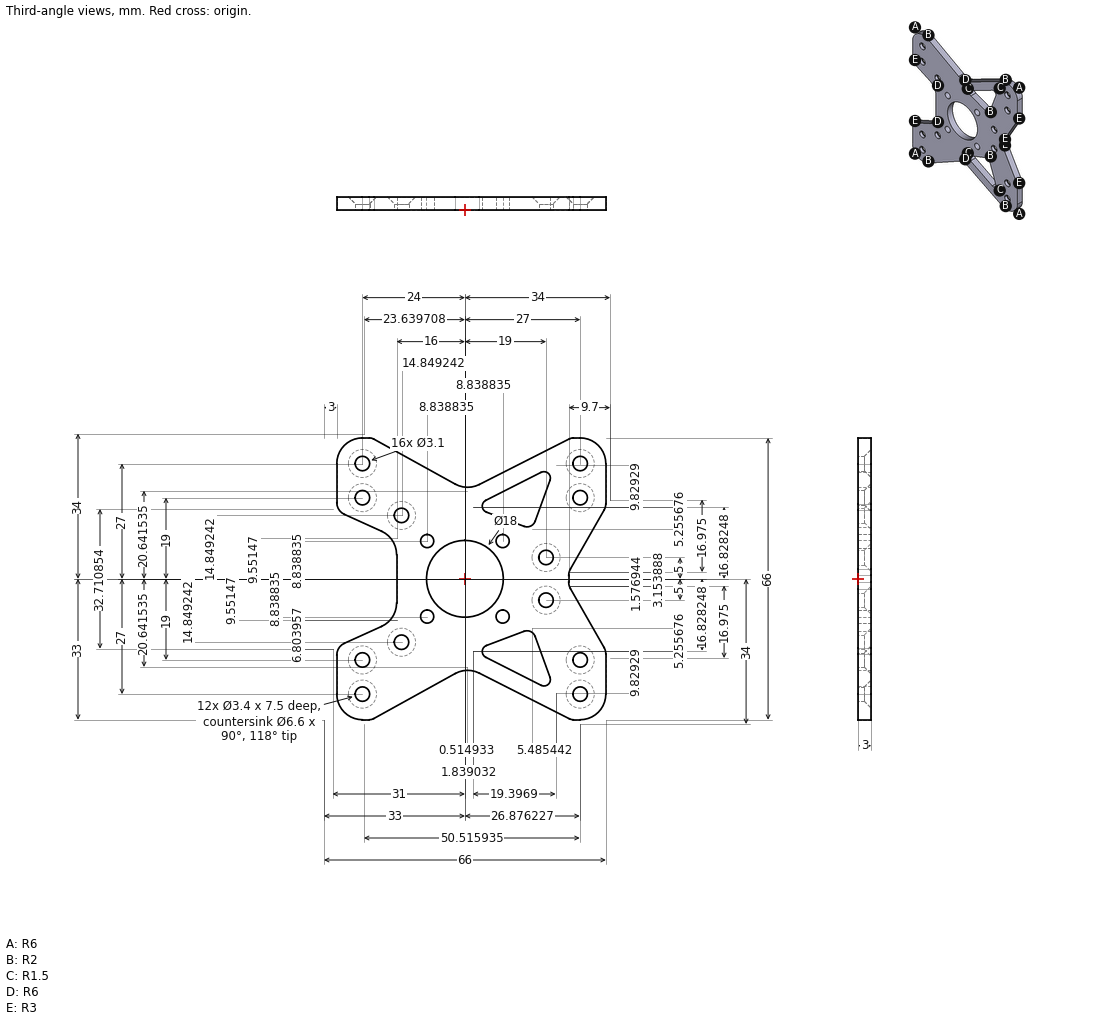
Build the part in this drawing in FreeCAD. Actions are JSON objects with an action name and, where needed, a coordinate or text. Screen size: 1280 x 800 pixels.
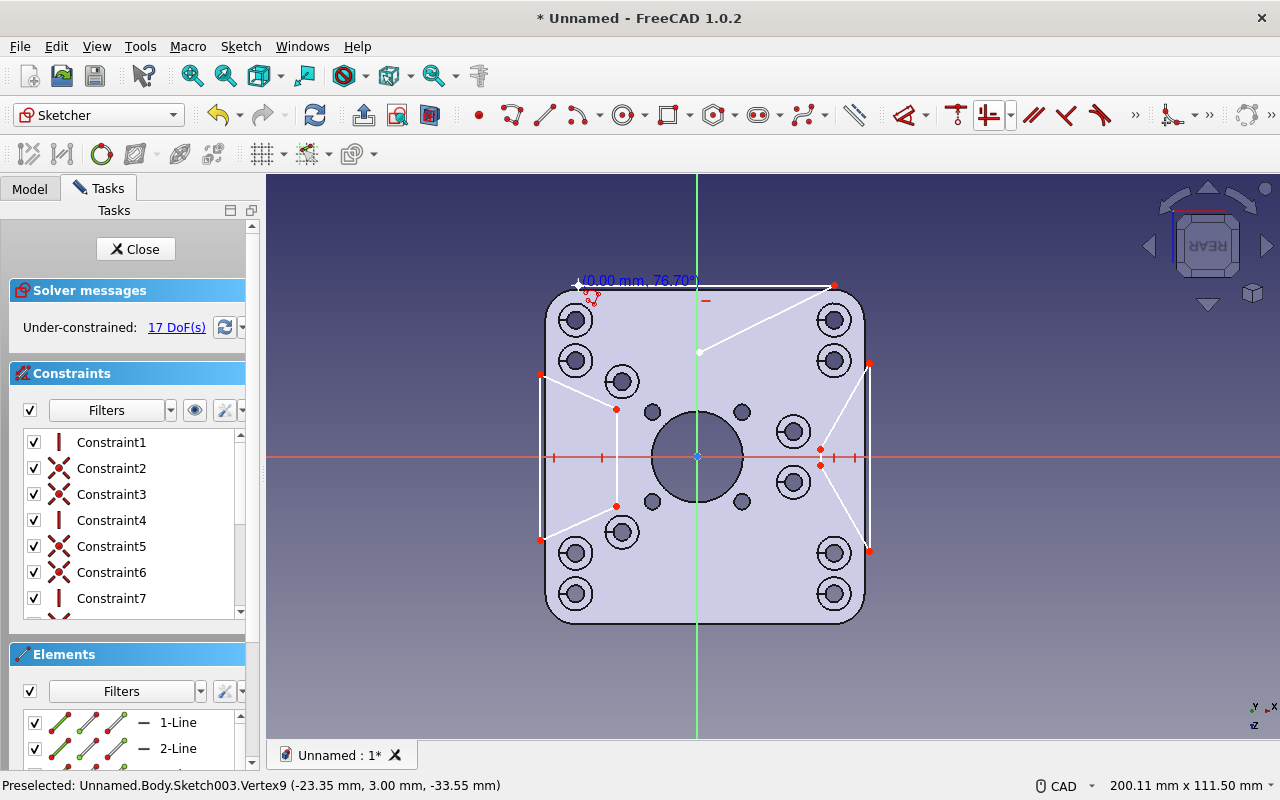
{"action": "scroll", "coordinate": [700, 352], "scroll_direction": "up", "scroll_amount": 10}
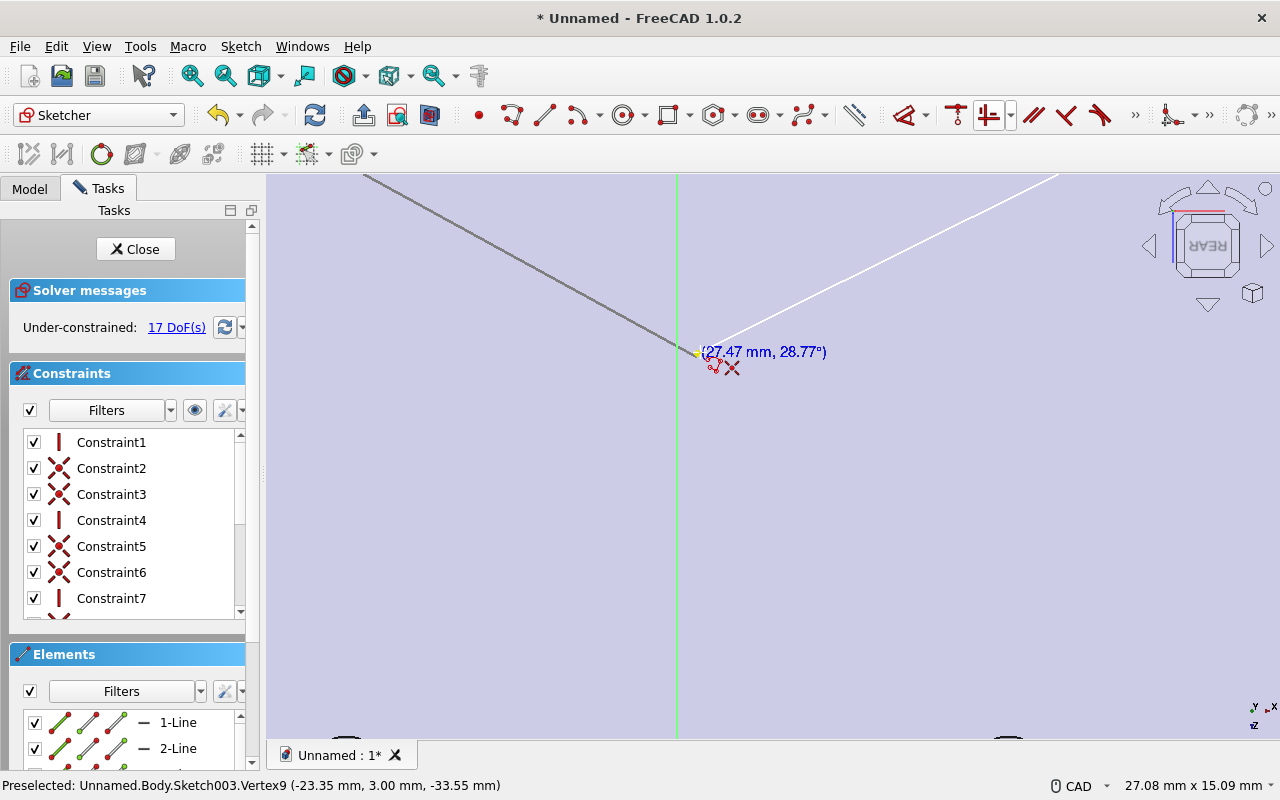
{"action": "left_click", "coordinate": [697, 354]}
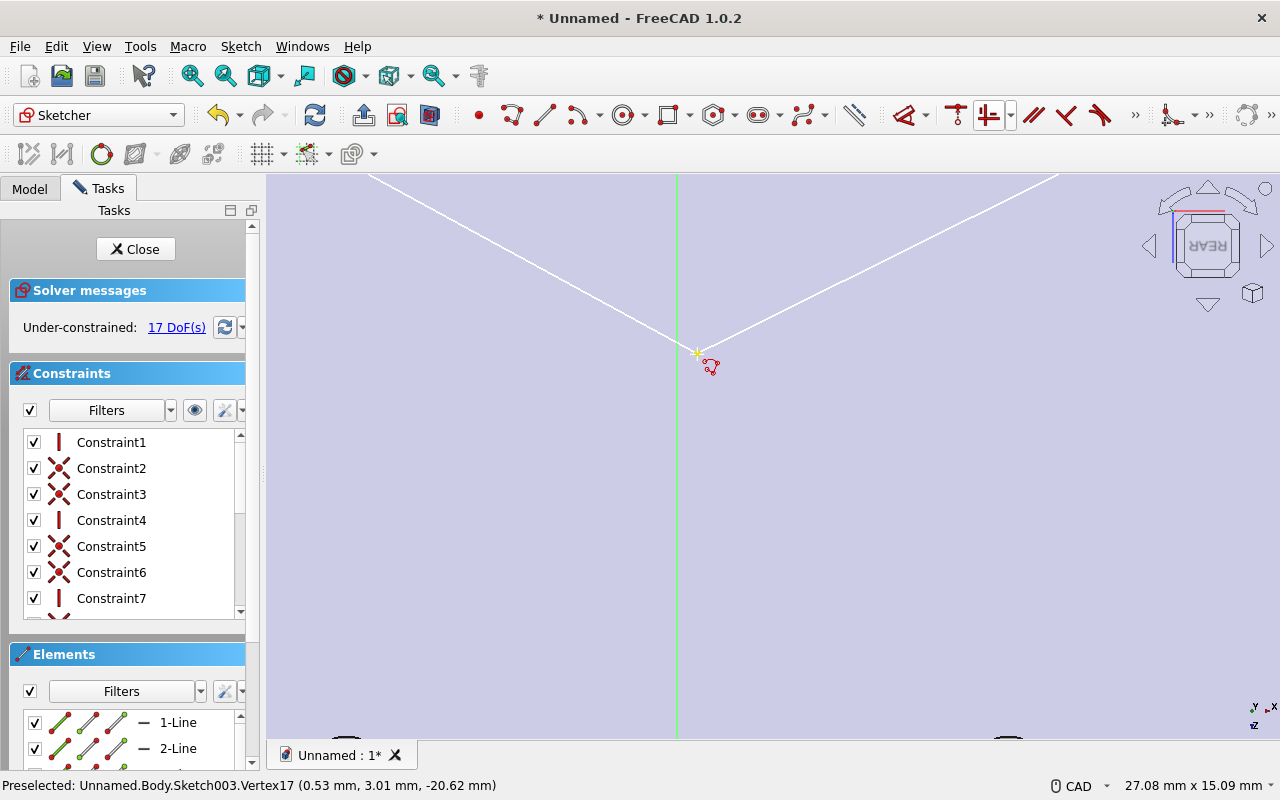
{"action": "scroll", "coordinate": [700, 352], "scroll_direction": "down", "scroll_amount": 10}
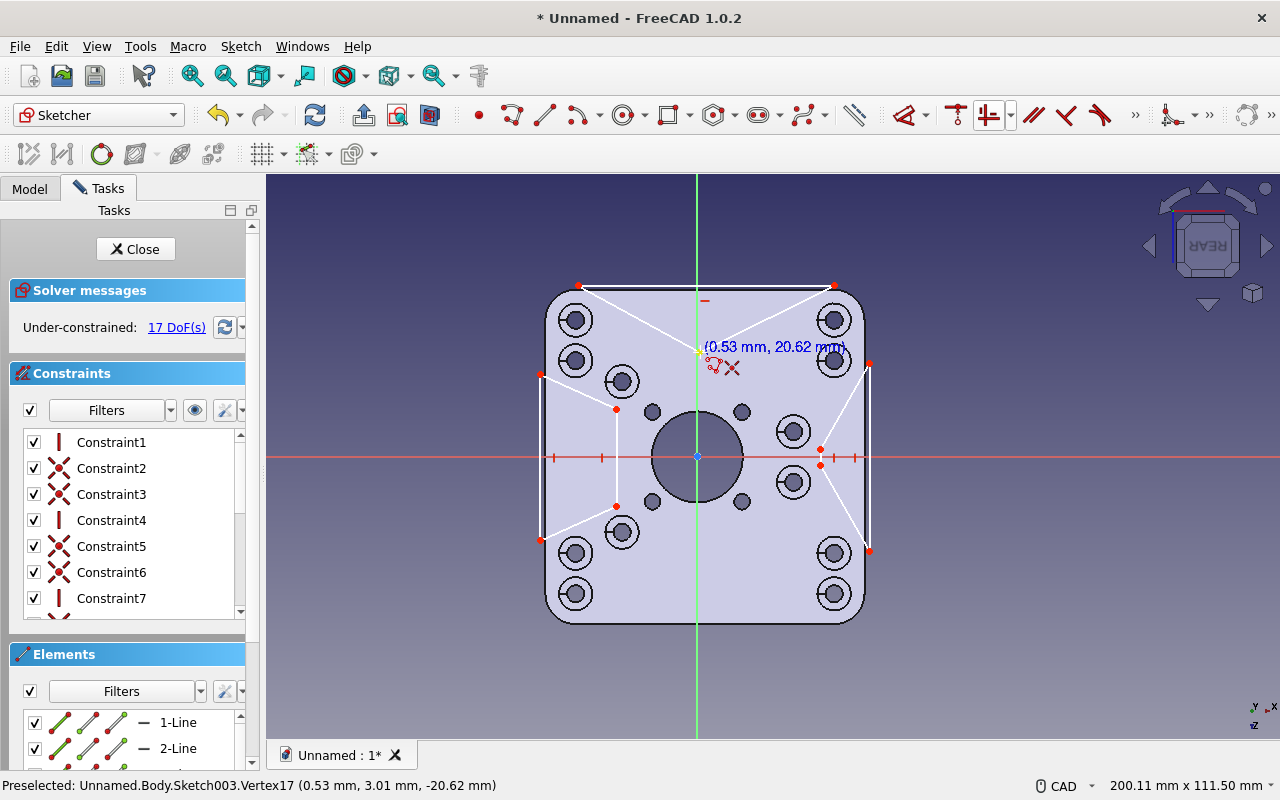
{"action": "scroll", "coordinate": [707, 372], "scroll_direction": "up", "scroll_amount": 3}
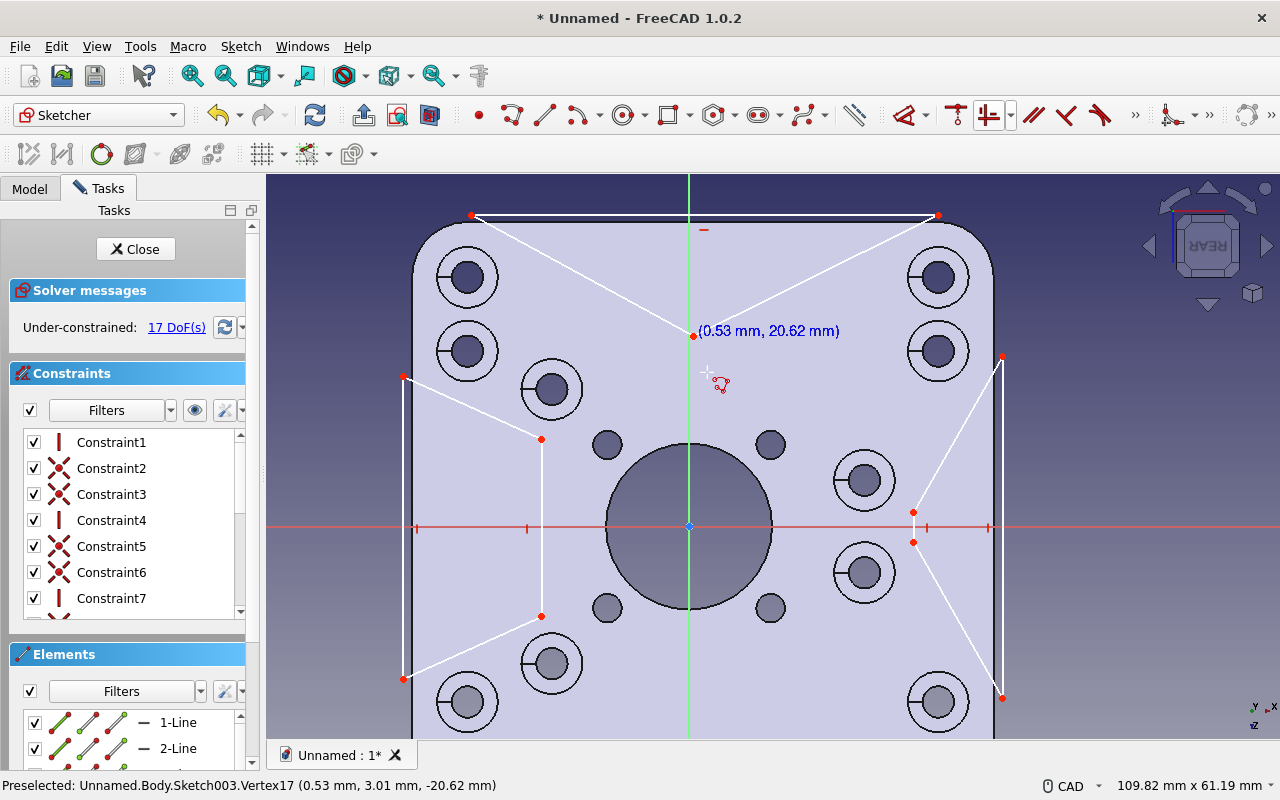
{"action": "left_click", "coordinate": [706, 371]}
{"action": "left_click", "coordinate": [834, 420]}
{"action": "left_click", "coordinate": [885, 280]}
{"action": "left_click", "coordinate": [706, 372]}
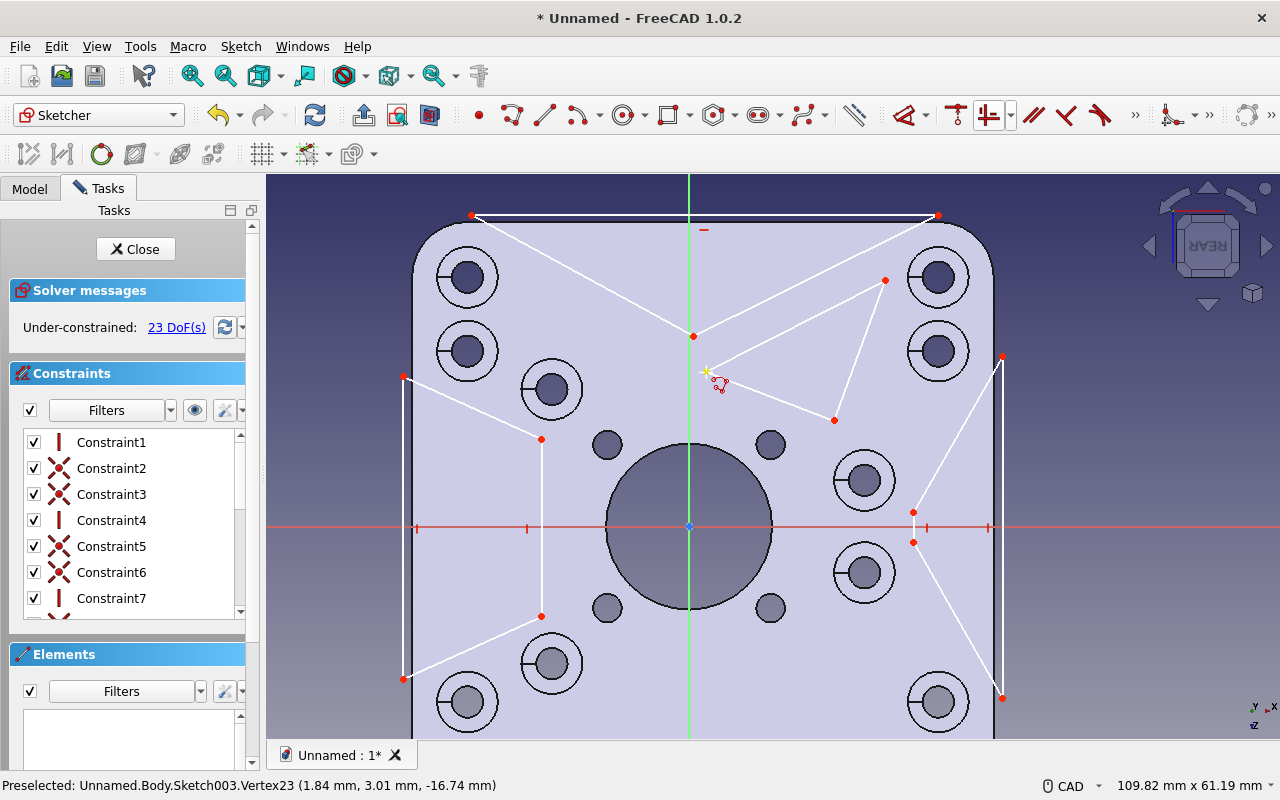
{"action": "left_click", "coordinate": [706, 682]}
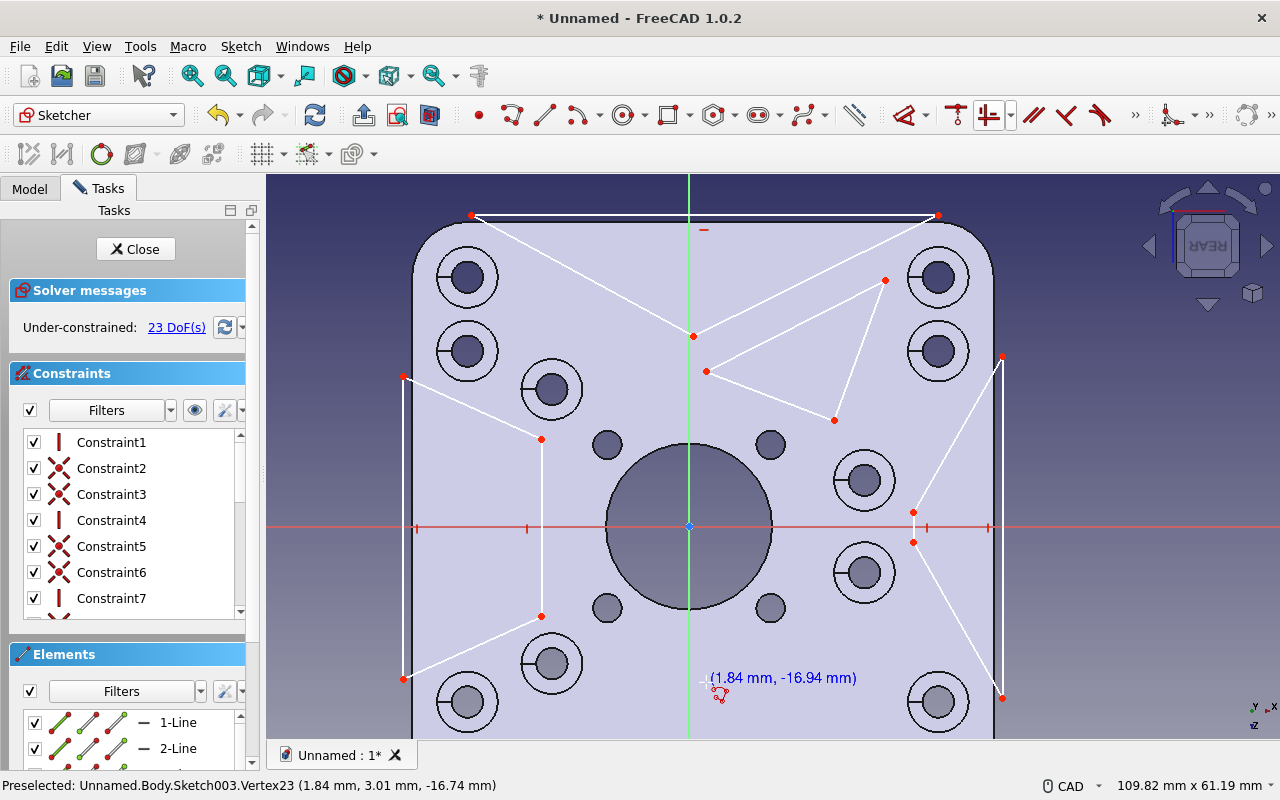
{"action": "scroll", "coordinate": [706, 371], "scroll_direction": "down", "scroll_amount": 3}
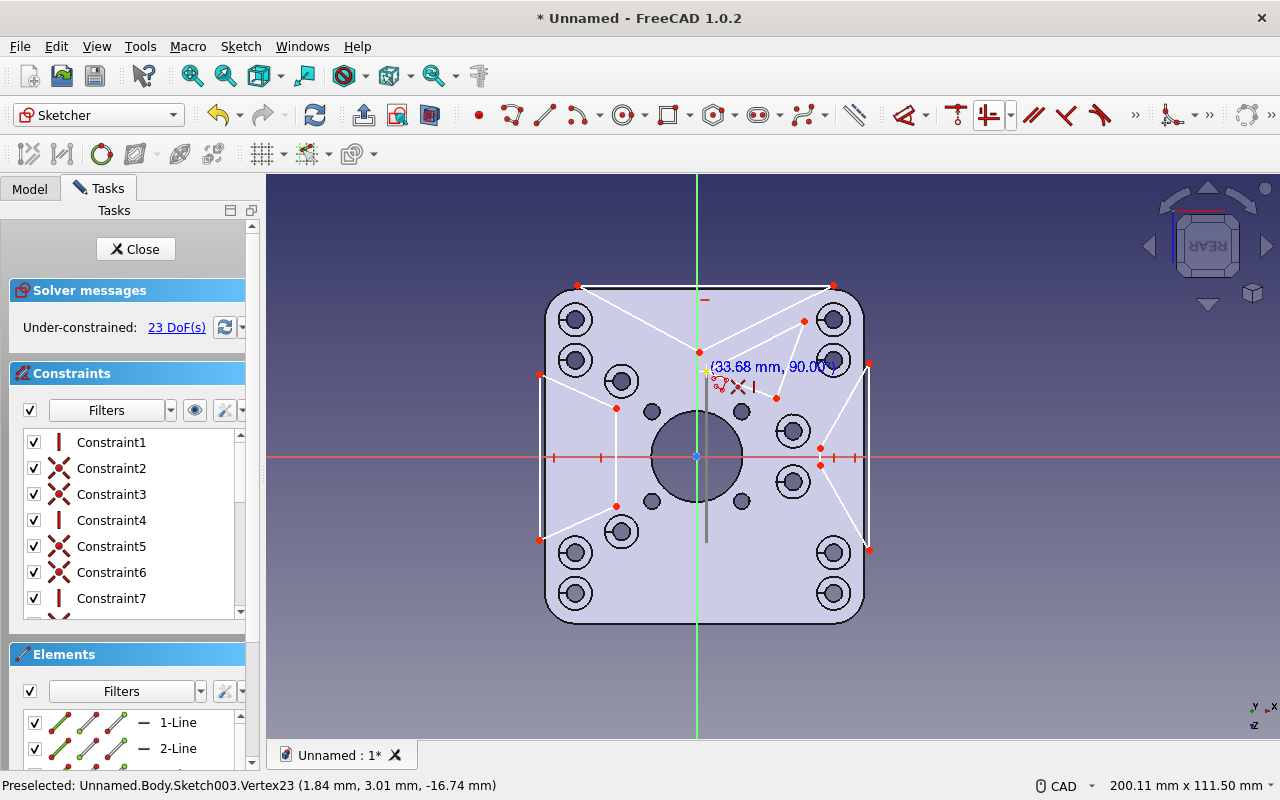
{"action": "left_click", "coordinate": [804, 592]}
{"action": "left_click", "coordinate": [777, 515]}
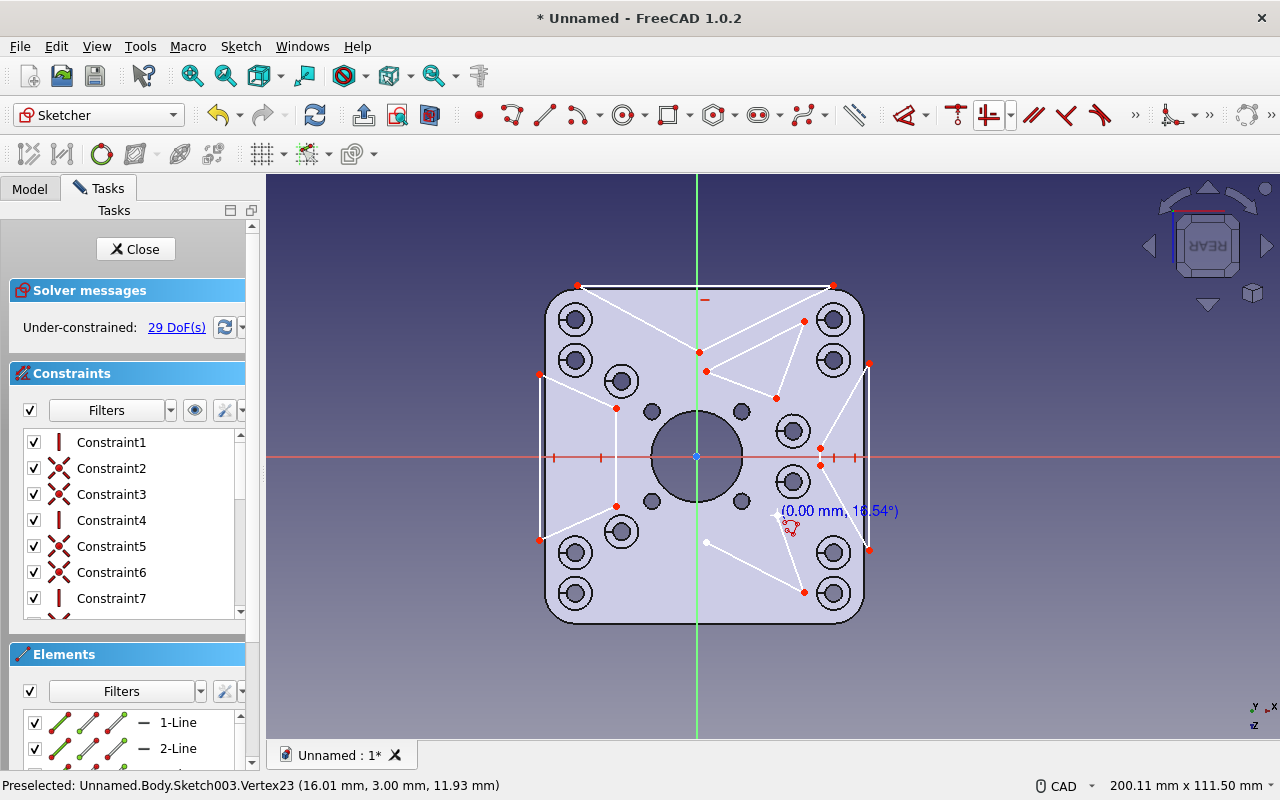
{"action": "scroll", "coordinate": [706, 542], "scroll_direction": "up", "scroll_amount": 3}